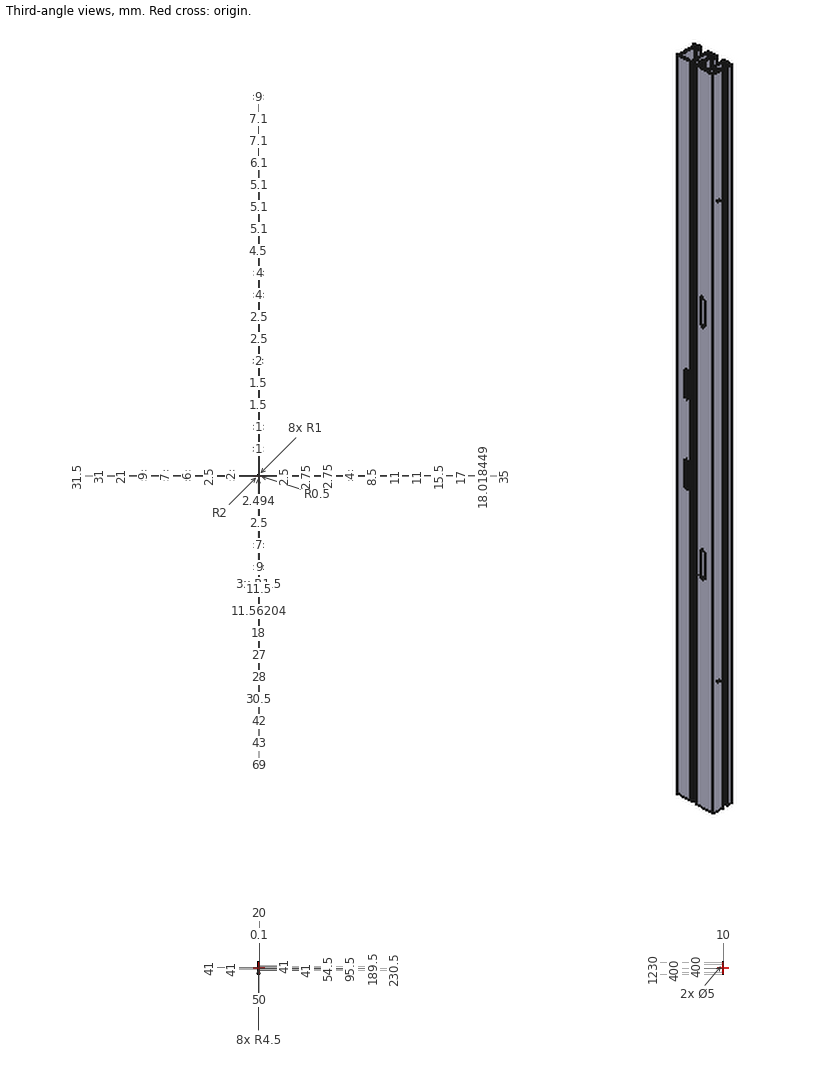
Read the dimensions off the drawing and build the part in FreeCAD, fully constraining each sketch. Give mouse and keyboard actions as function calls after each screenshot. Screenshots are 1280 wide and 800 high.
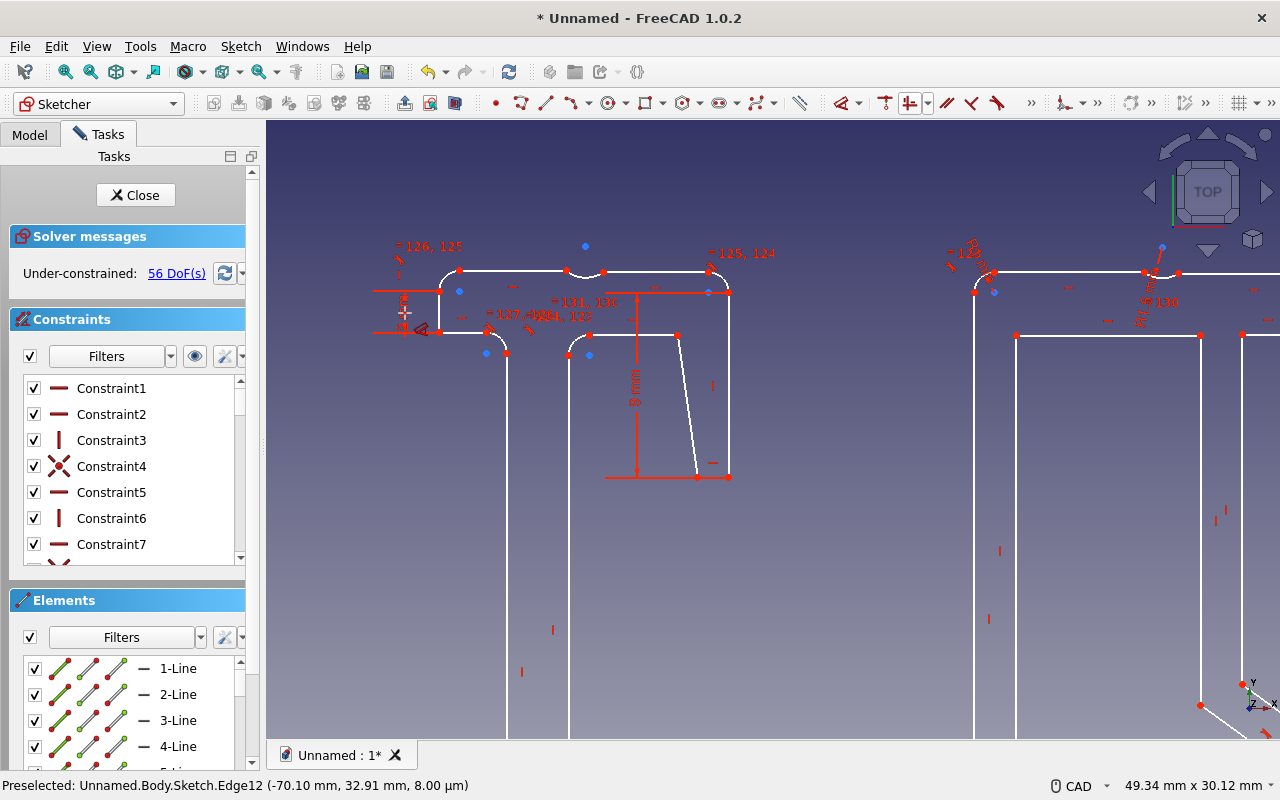
click(453, 333)
click(479, 299)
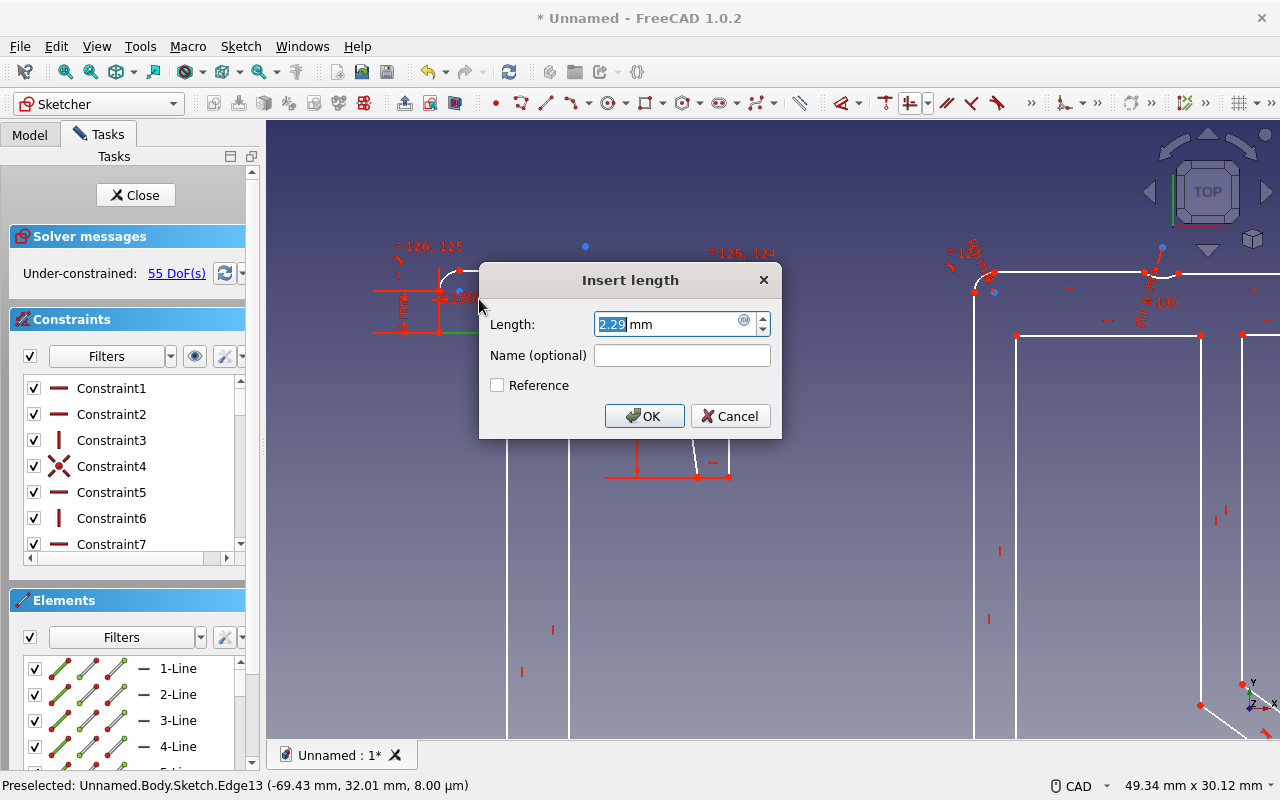
text(2)
key(Return)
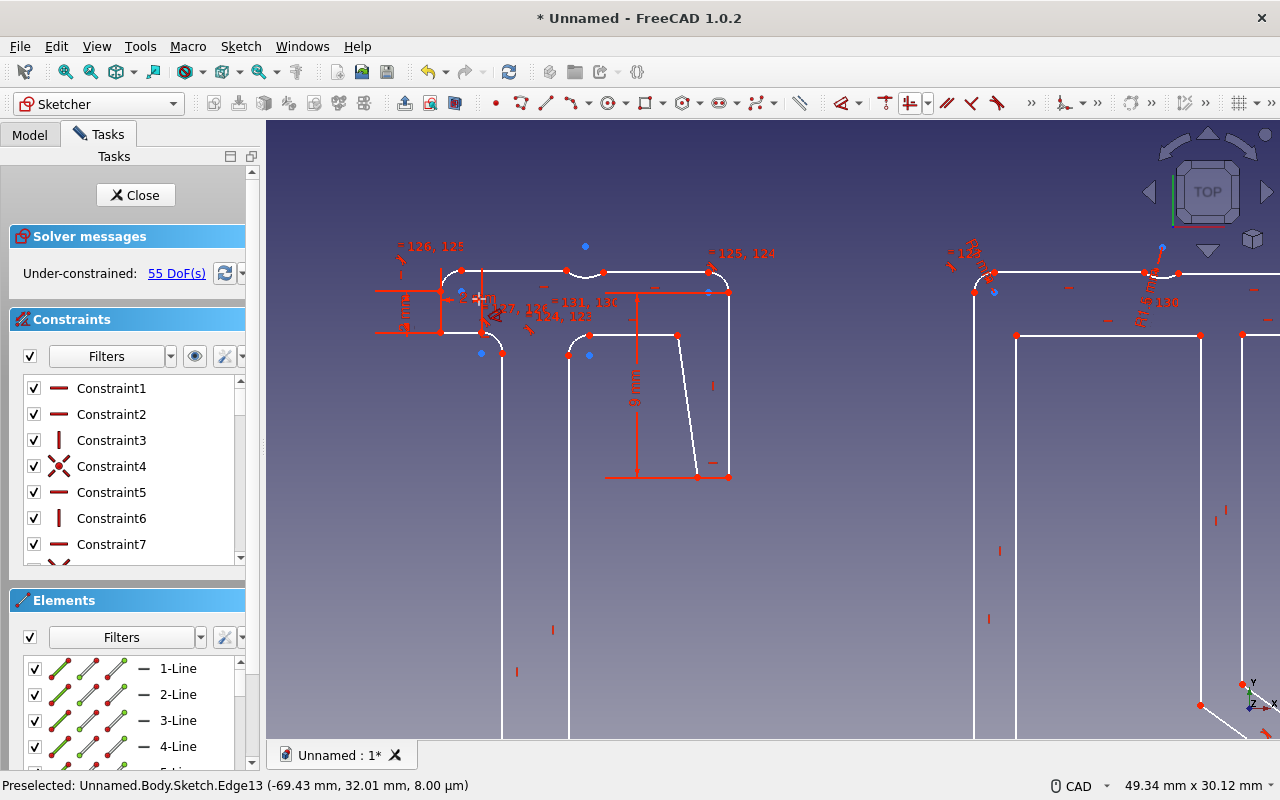
scroll(439, 312, down, 5)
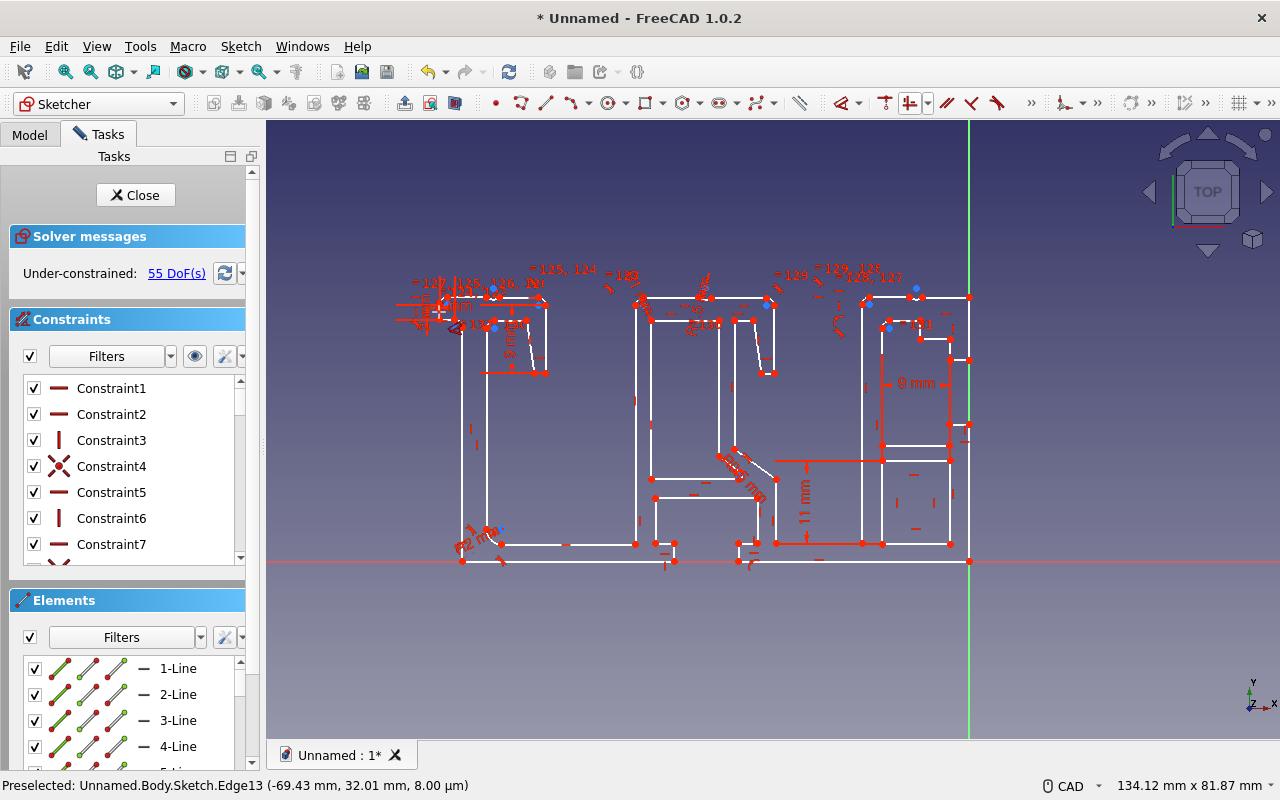
click(656, 530)
click(622, 521)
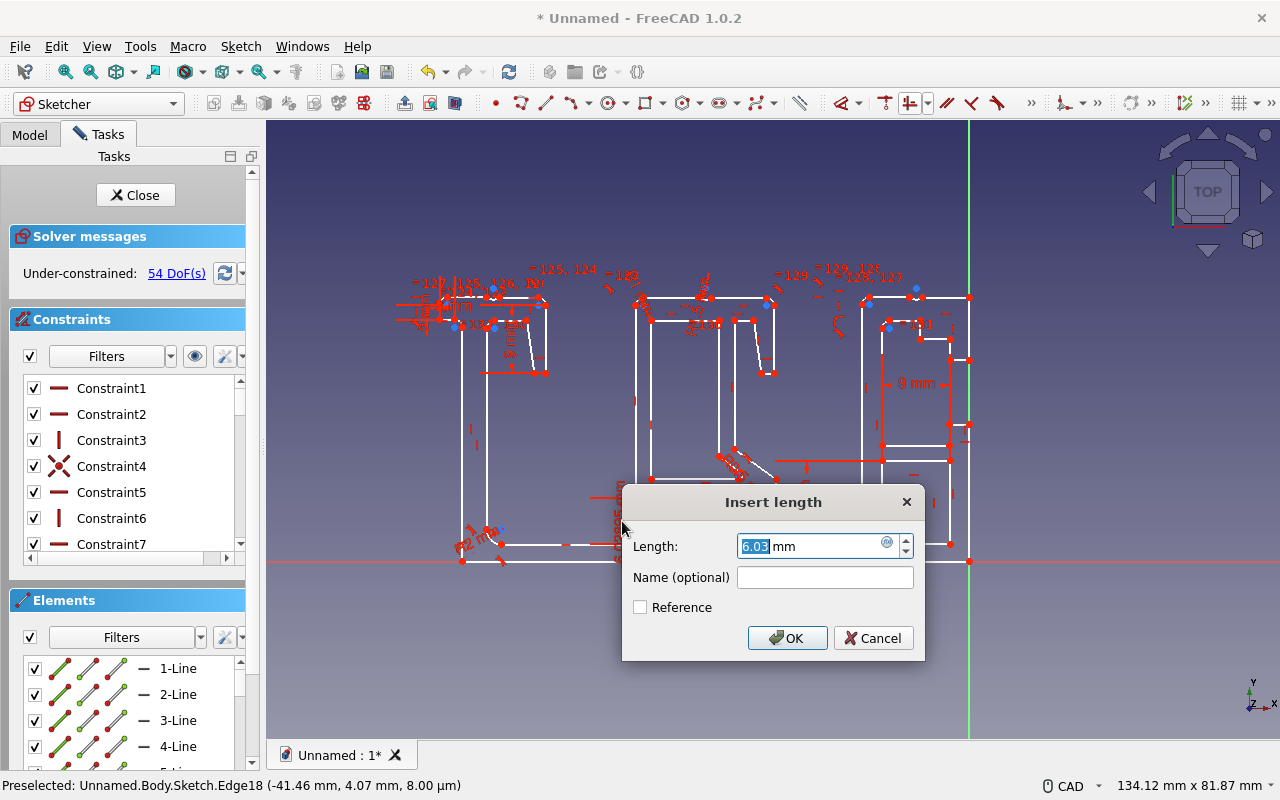
text(6)
key(Return)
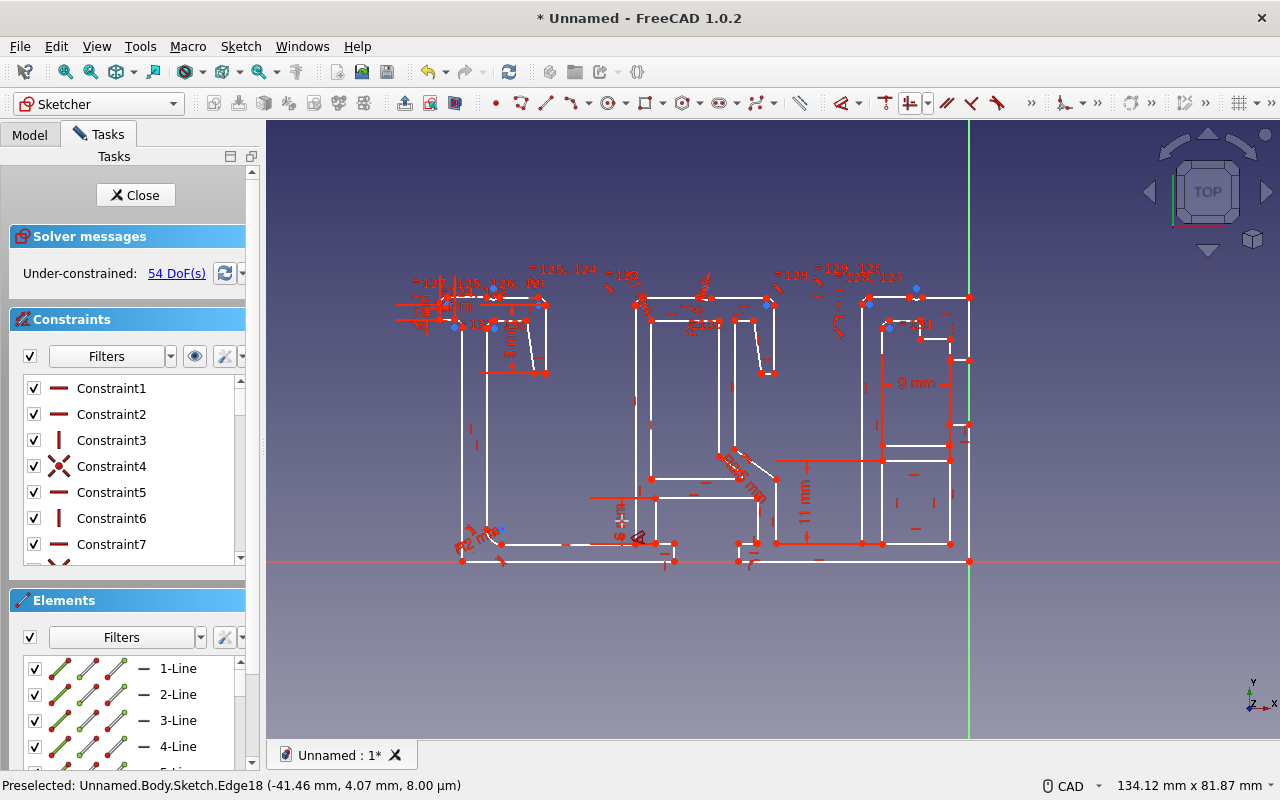
click(758, 512)
click(792, 521)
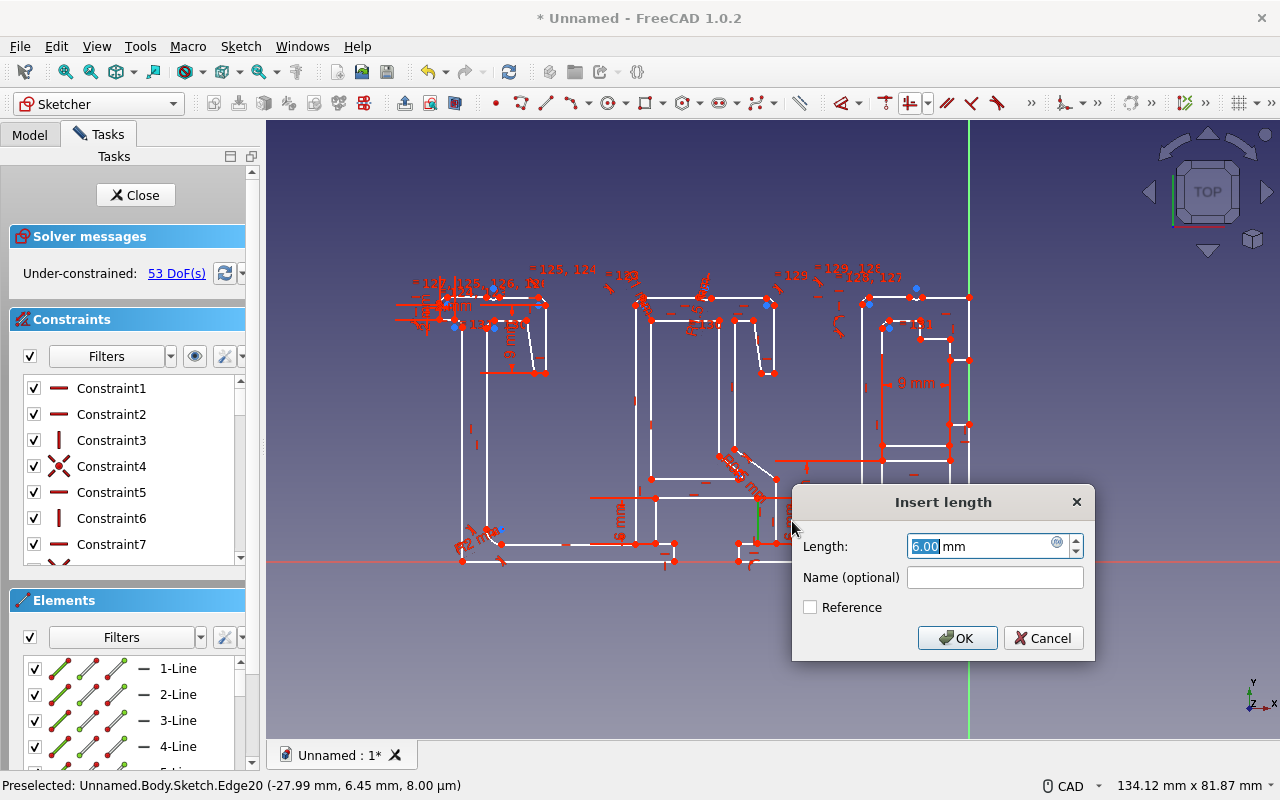
text(6)
key(Return)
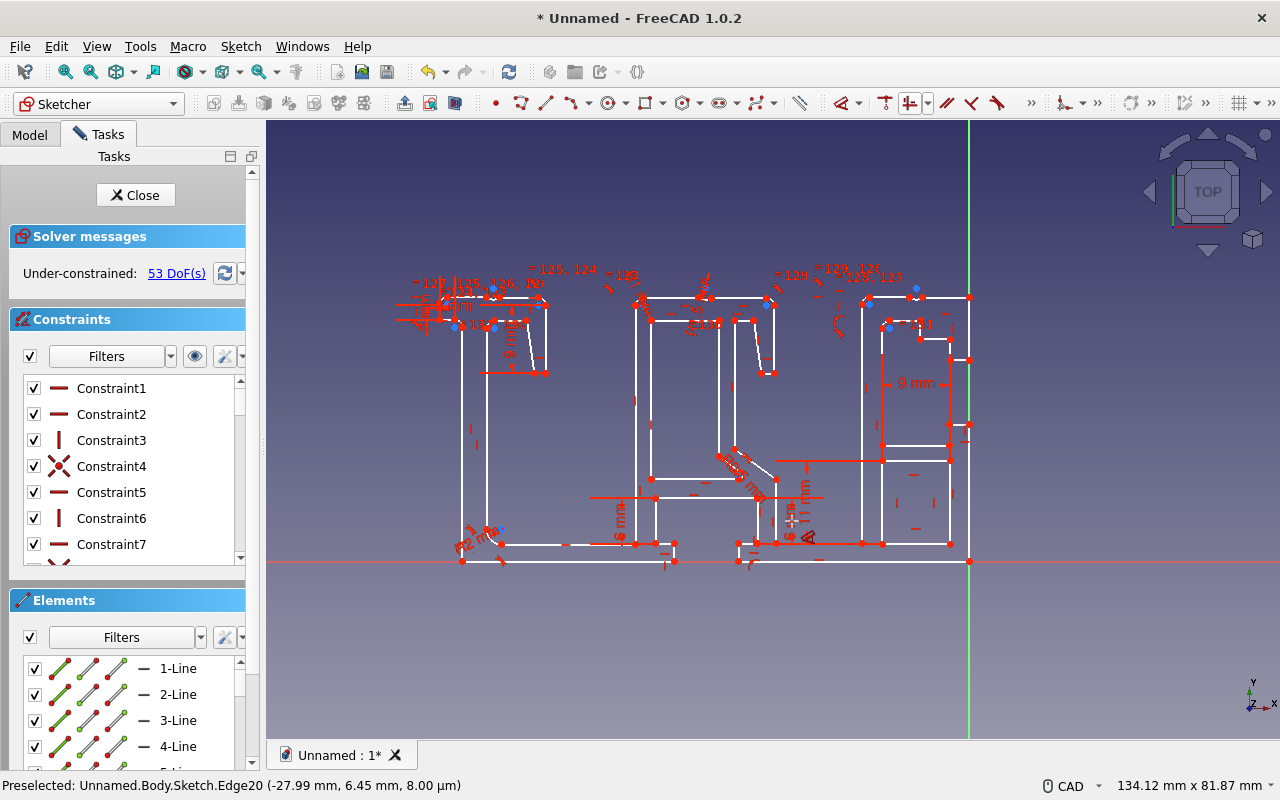
click(930, 446)
click(916, 480)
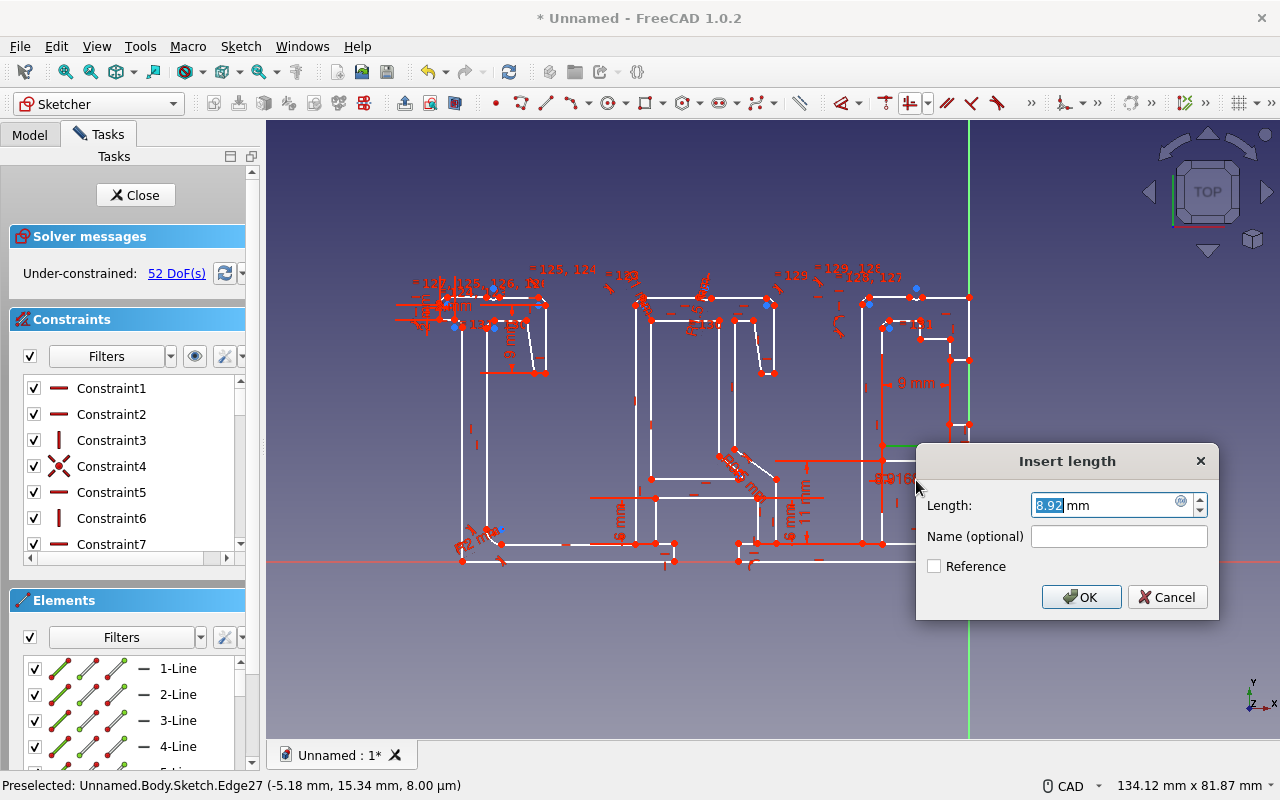
text(9)
key(Return)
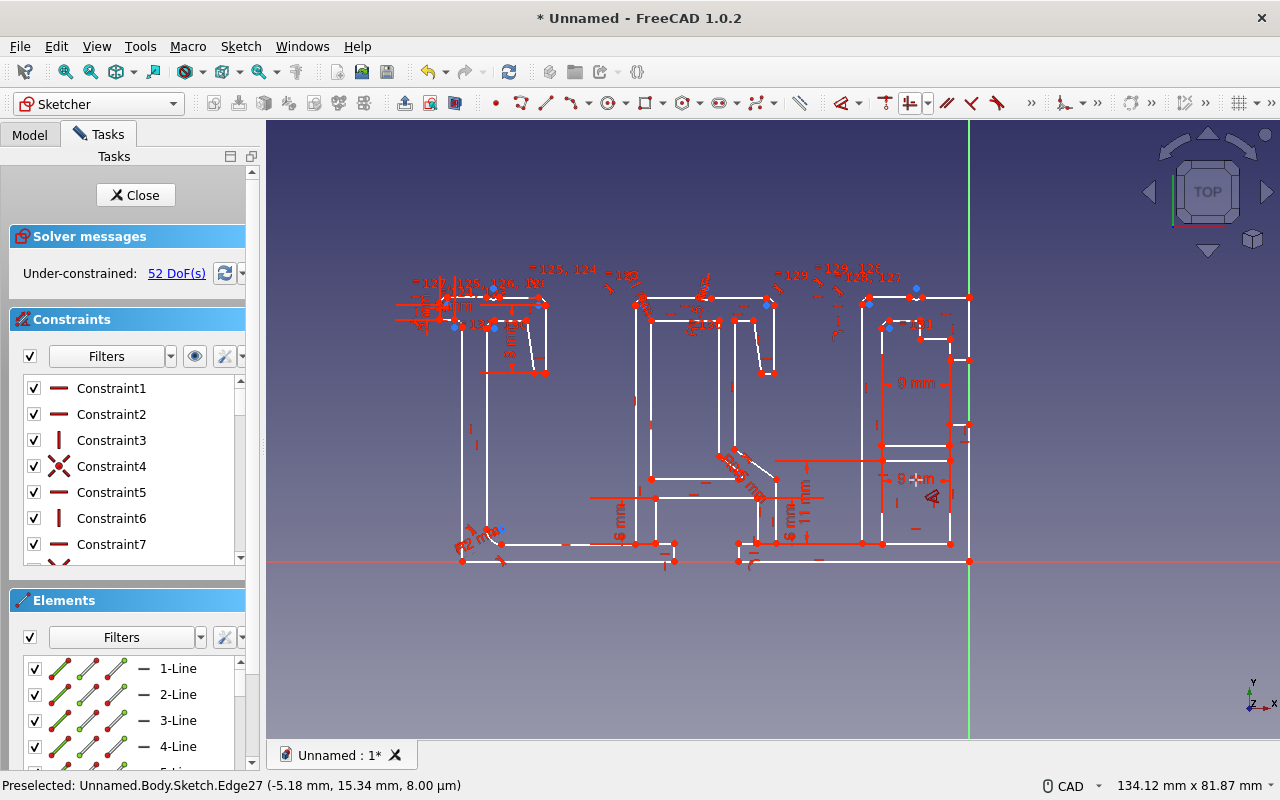
scroll(899, 321, up, 3)